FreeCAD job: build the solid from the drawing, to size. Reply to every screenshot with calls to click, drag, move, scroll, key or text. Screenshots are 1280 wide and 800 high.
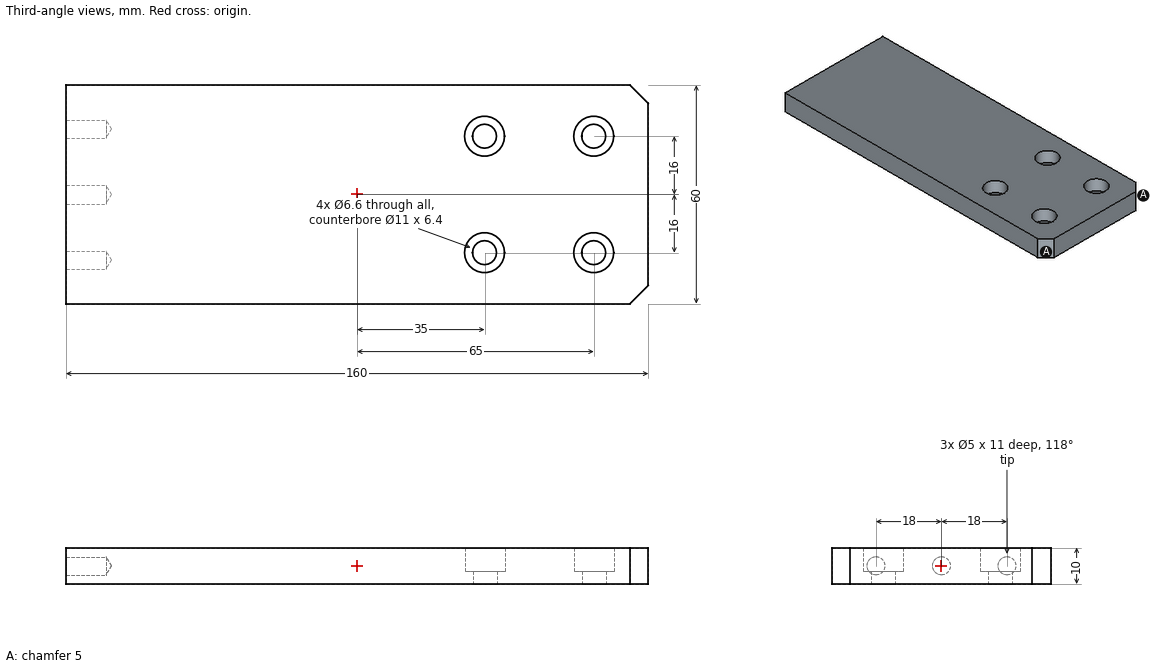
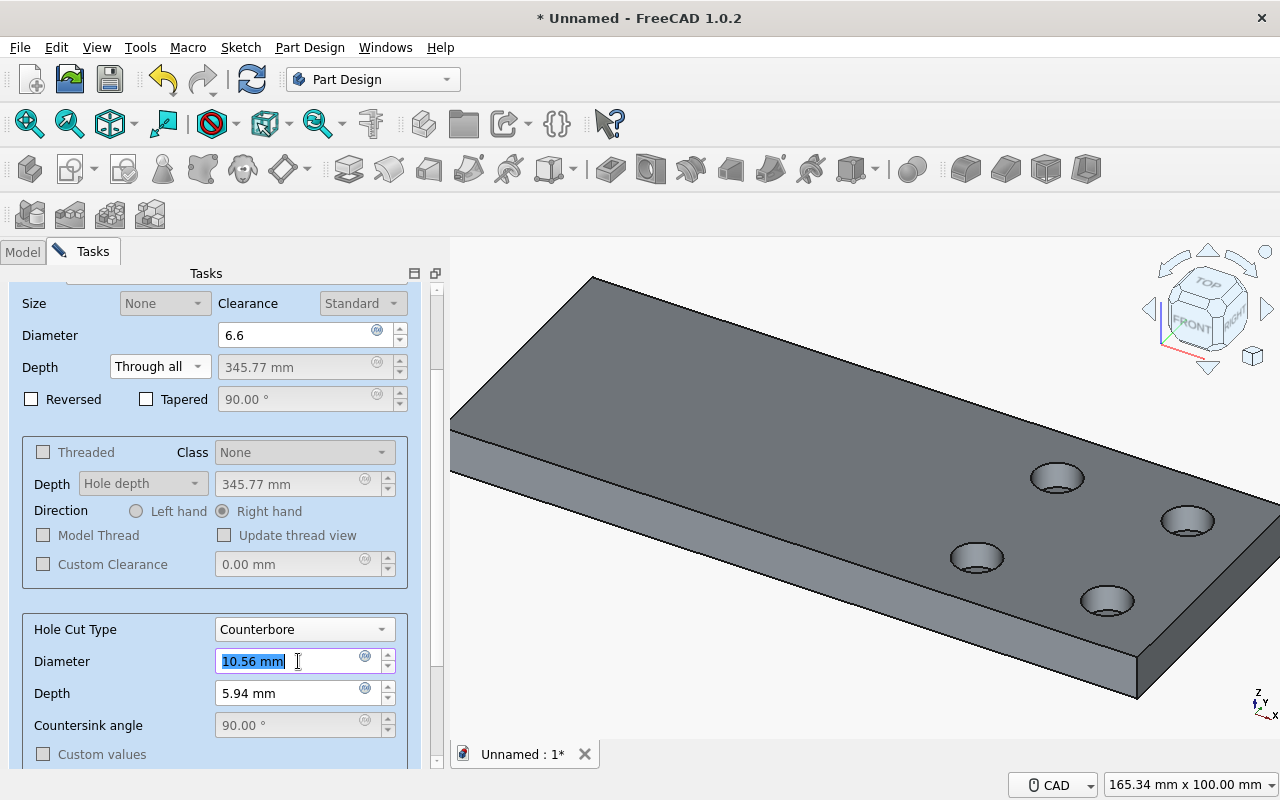
text(11)
key(Tab)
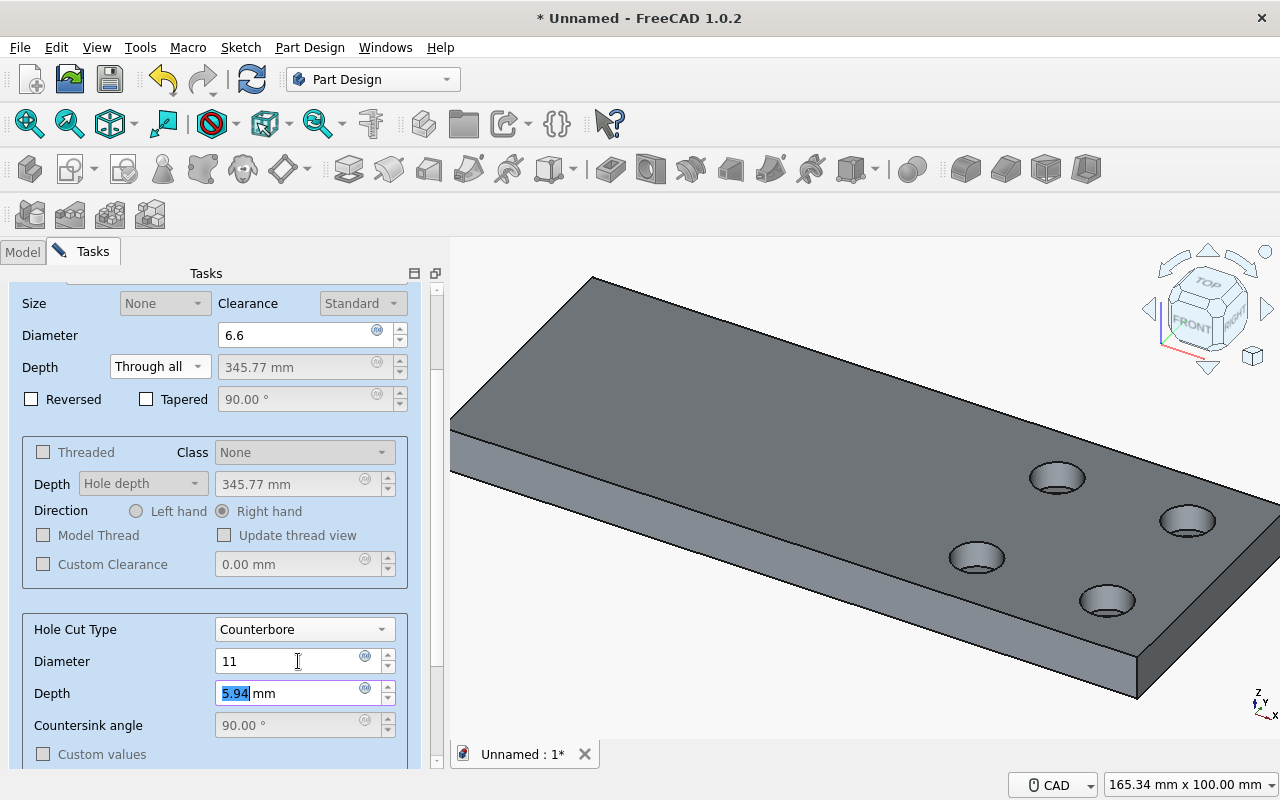
text(6.4)
key(Tab)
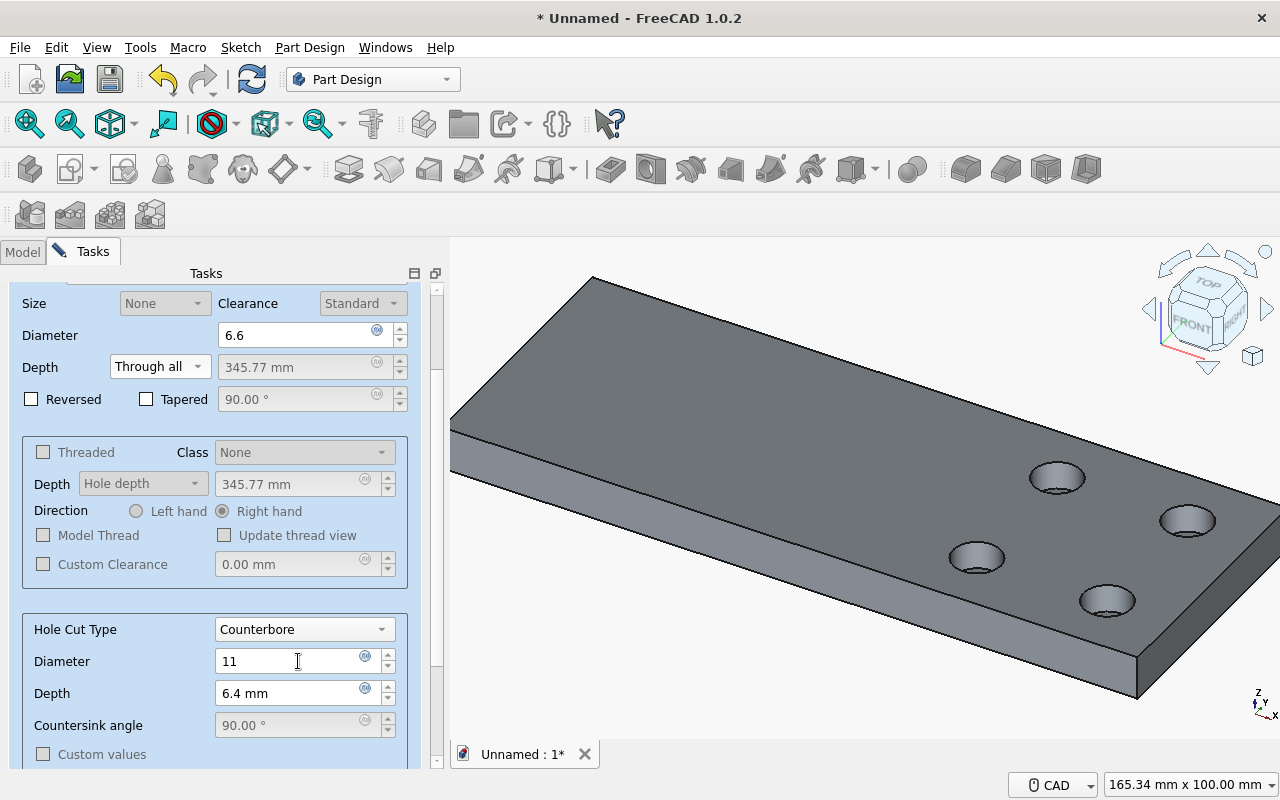
scroll(437, 526, up, 3)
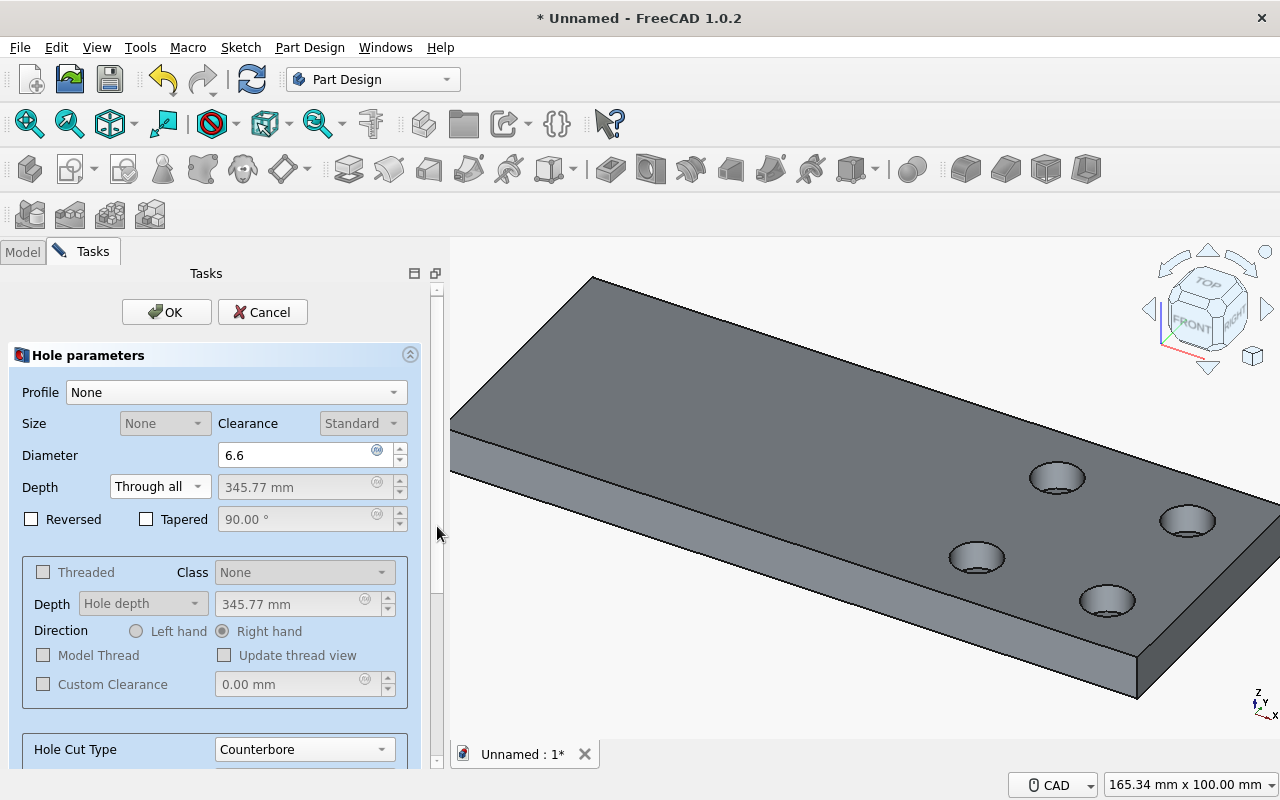
click(167, 312)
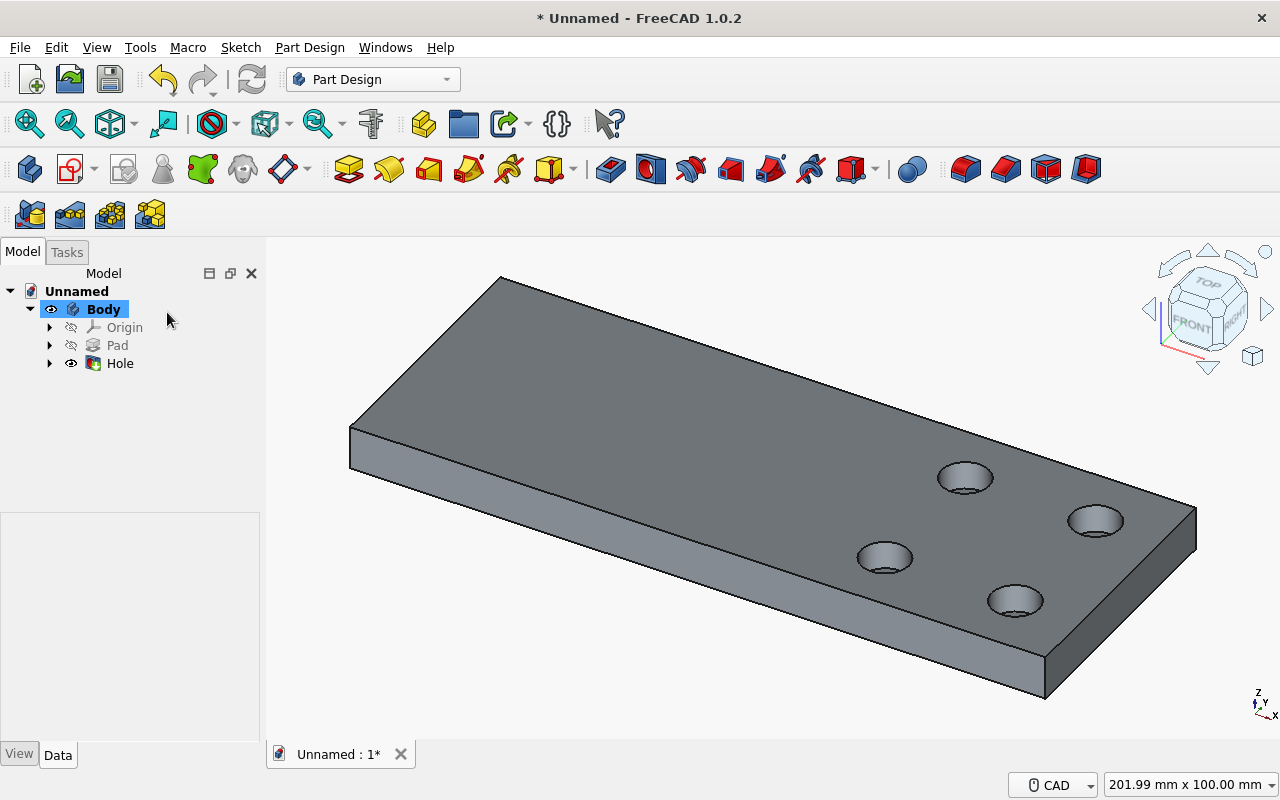
click(1045, 677)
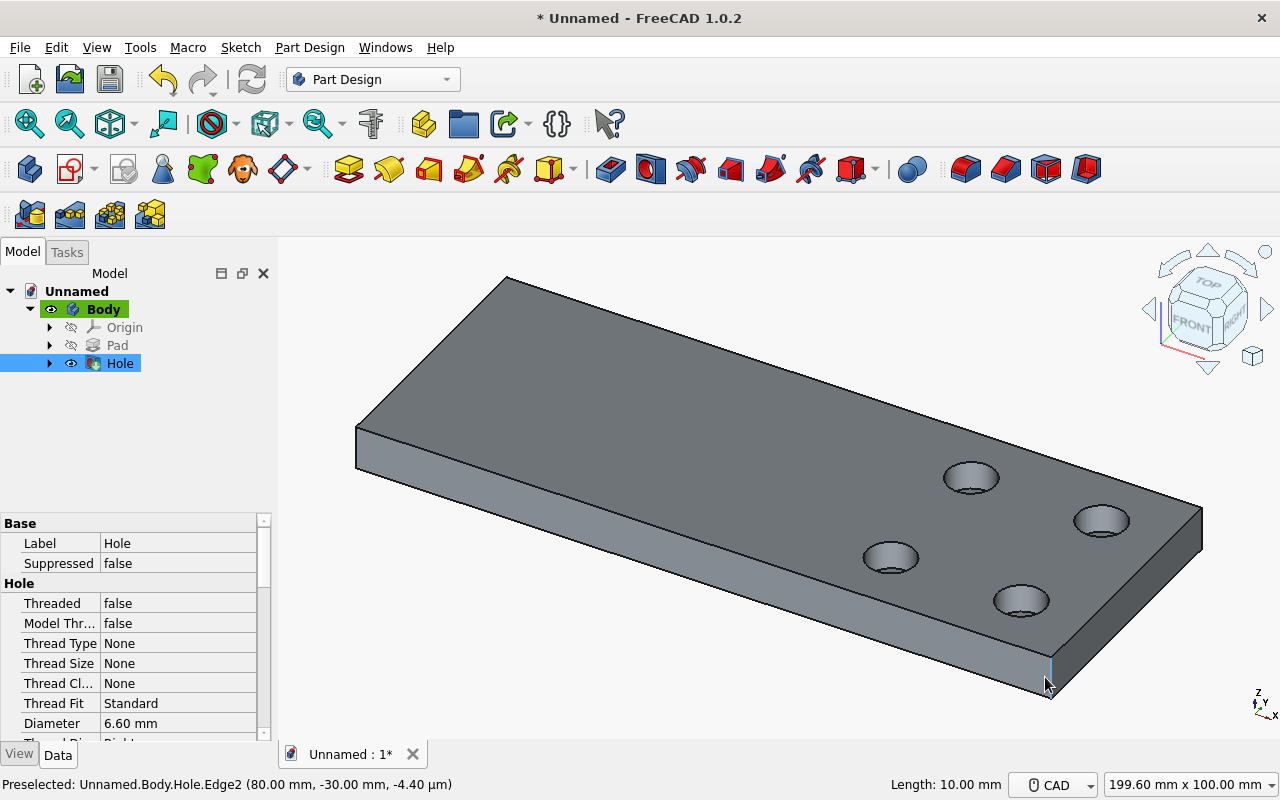
key(0)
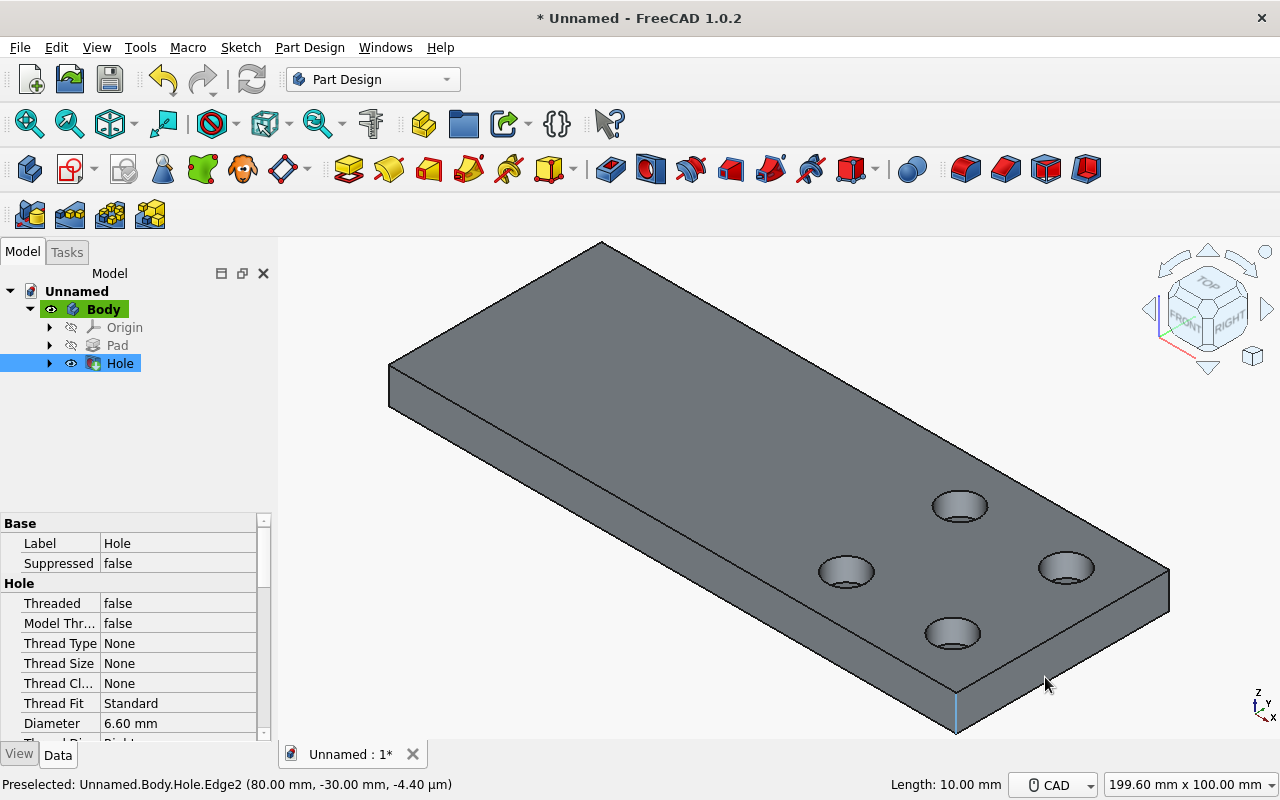
key(2)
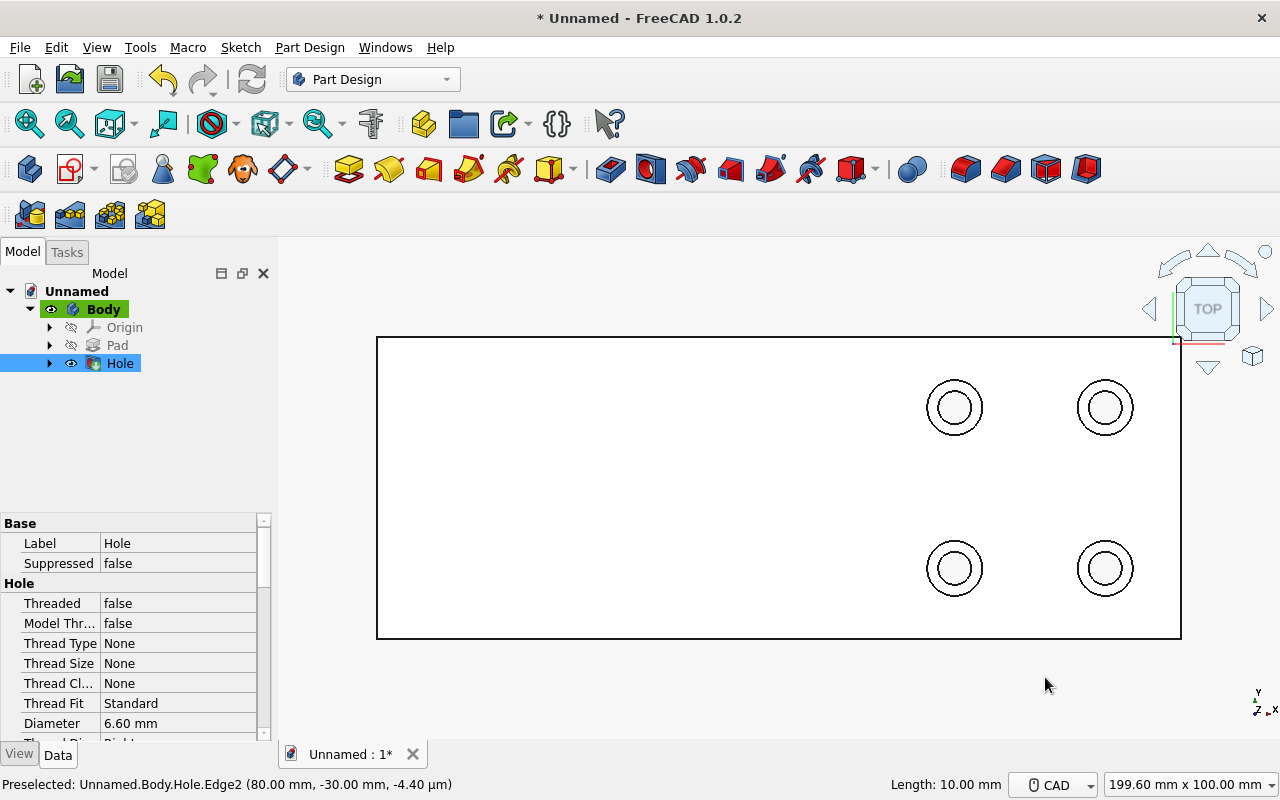
key(1)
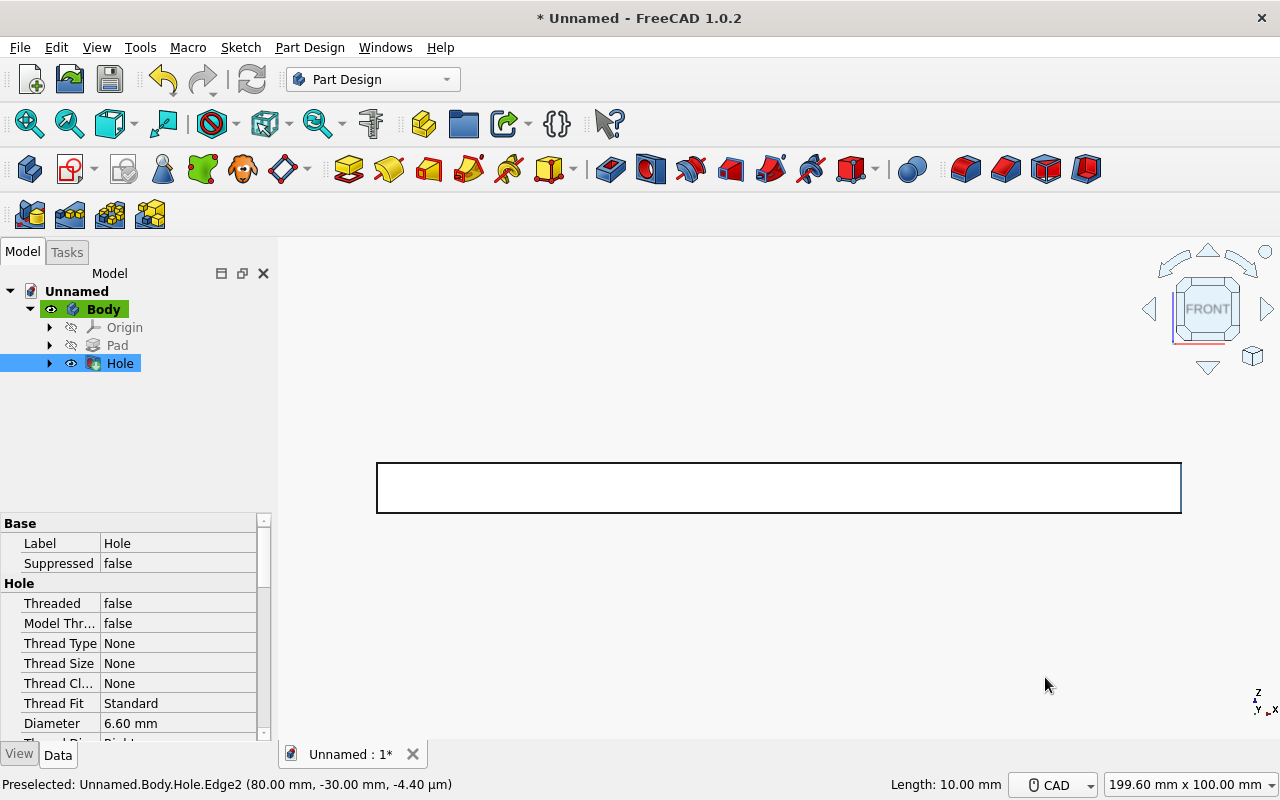
key(3)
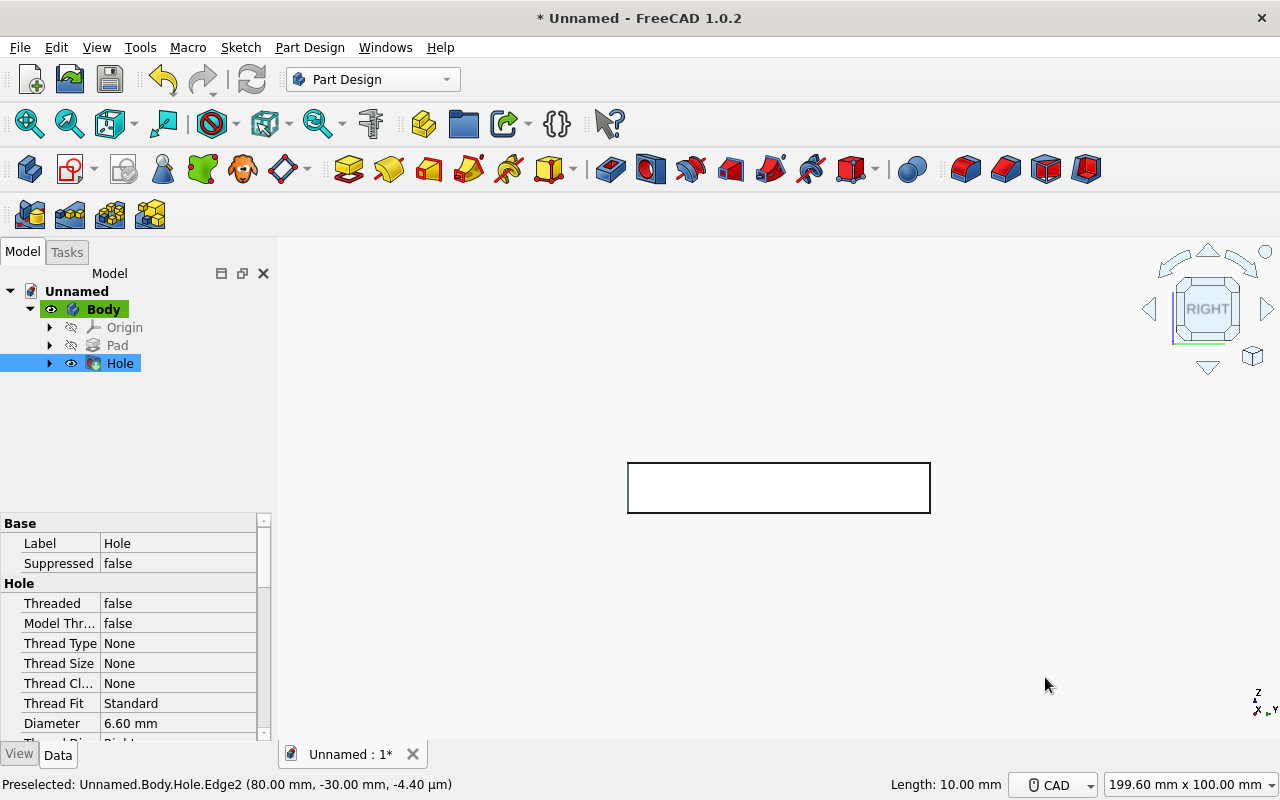
key(v)
key(f)